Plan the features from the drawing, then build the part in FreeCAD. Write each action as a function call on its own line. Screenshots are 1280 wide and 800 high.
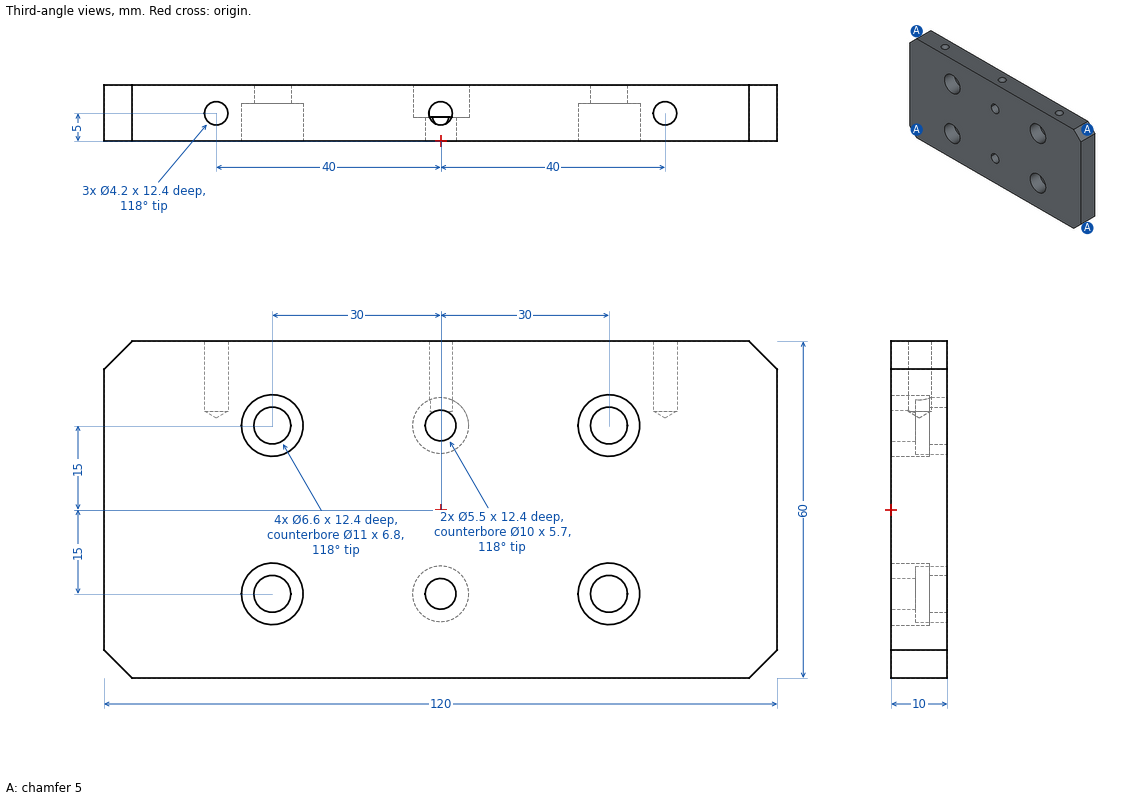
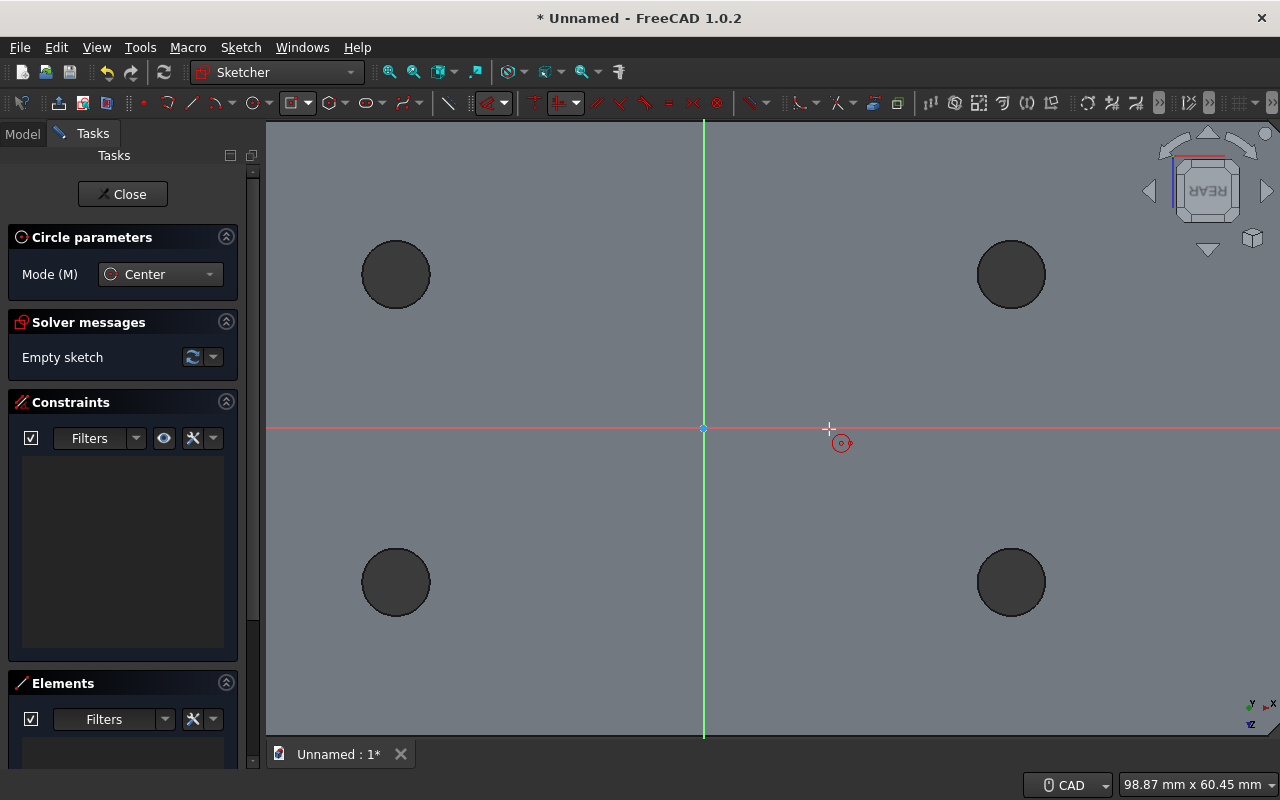
click(704, 582)
move(724, 562)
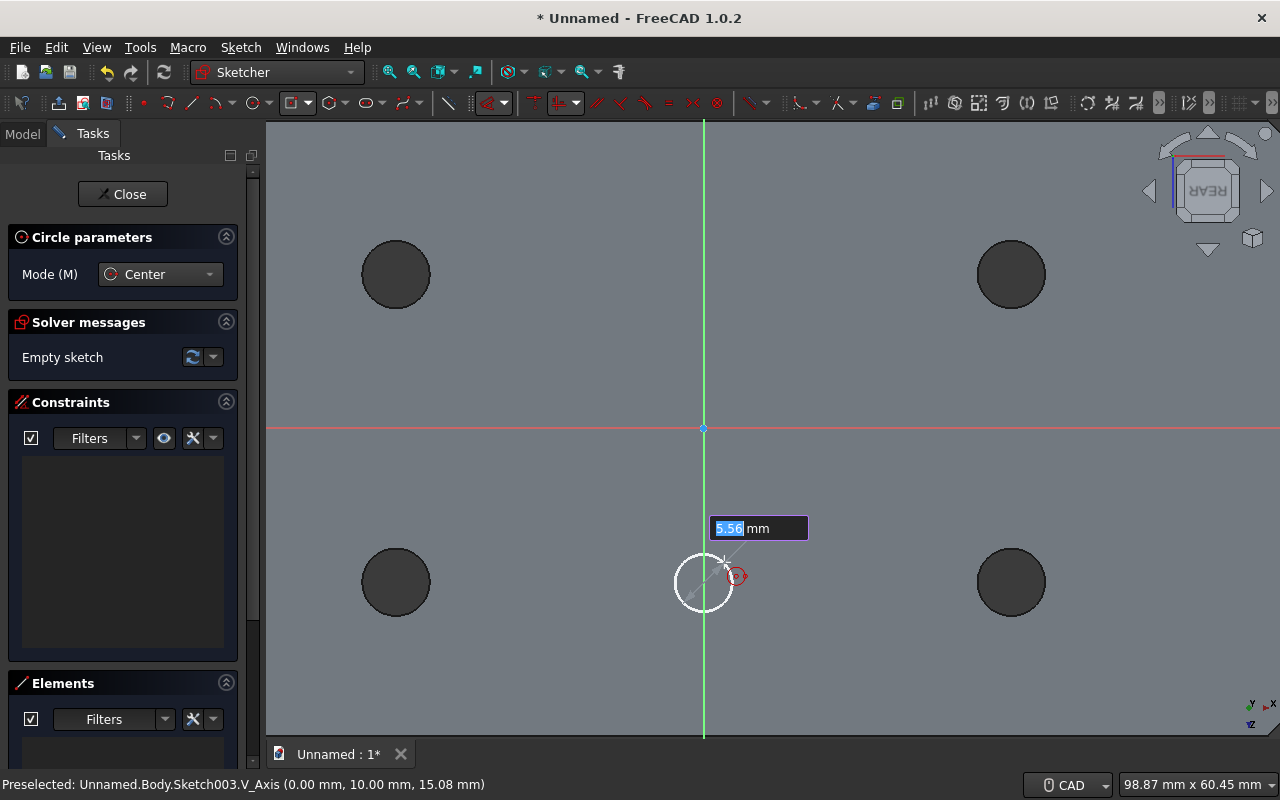
text(5.5)
key(Return)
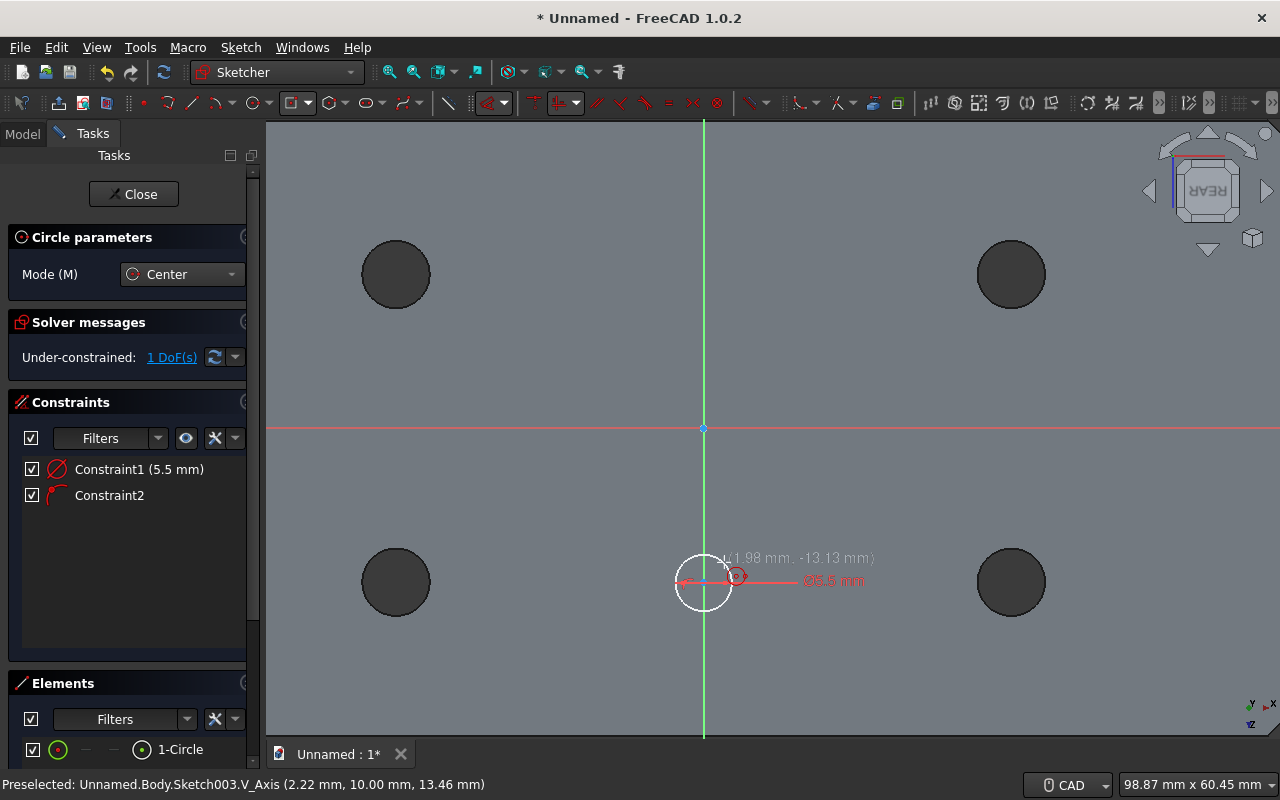
click(704, 275)
move(724, 255)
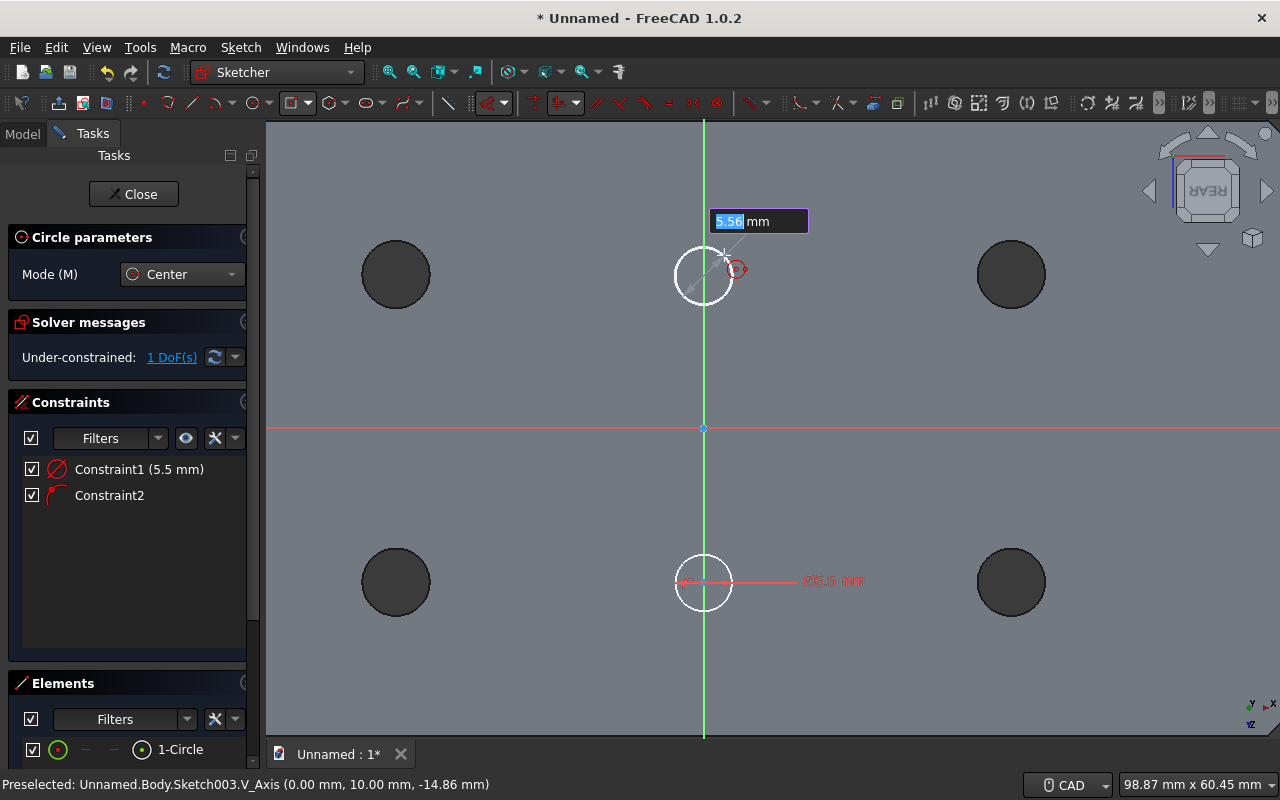
text(5.5)
key(Return)
key(Escape)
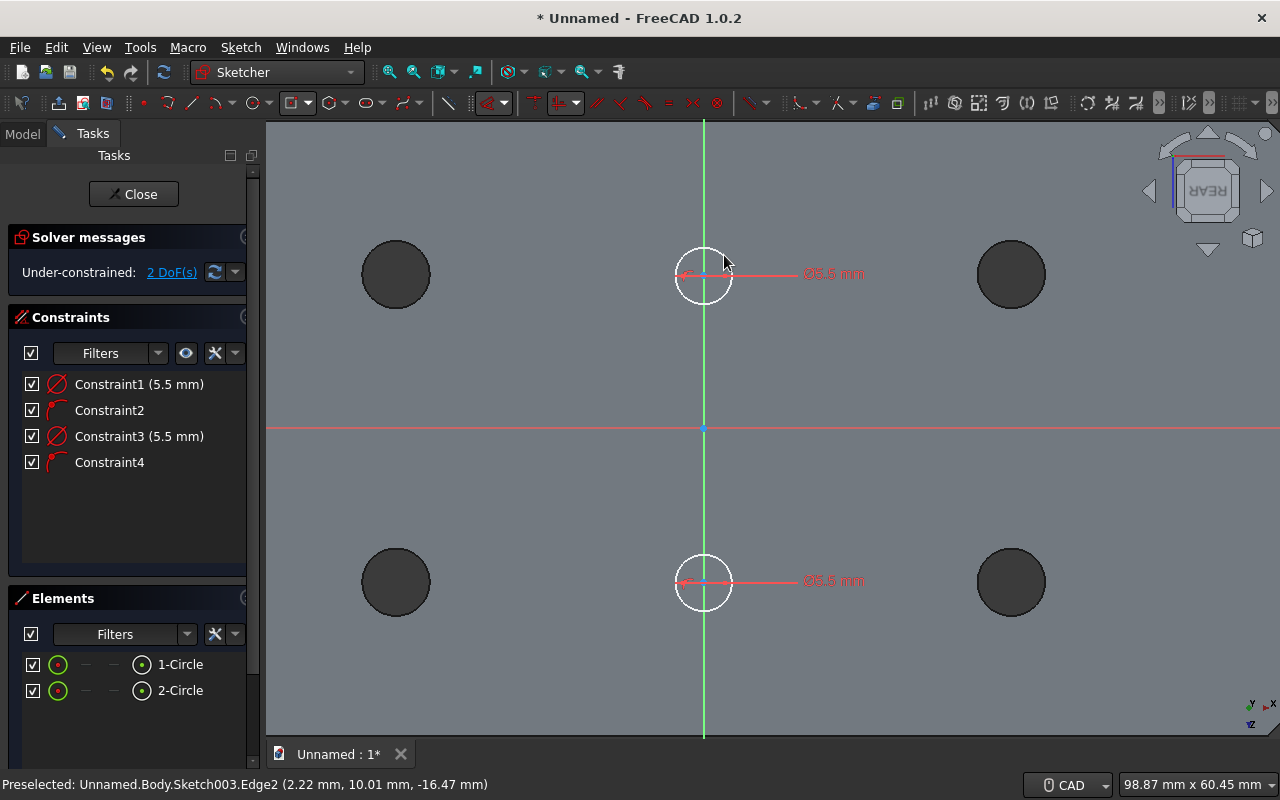
click(704, 583)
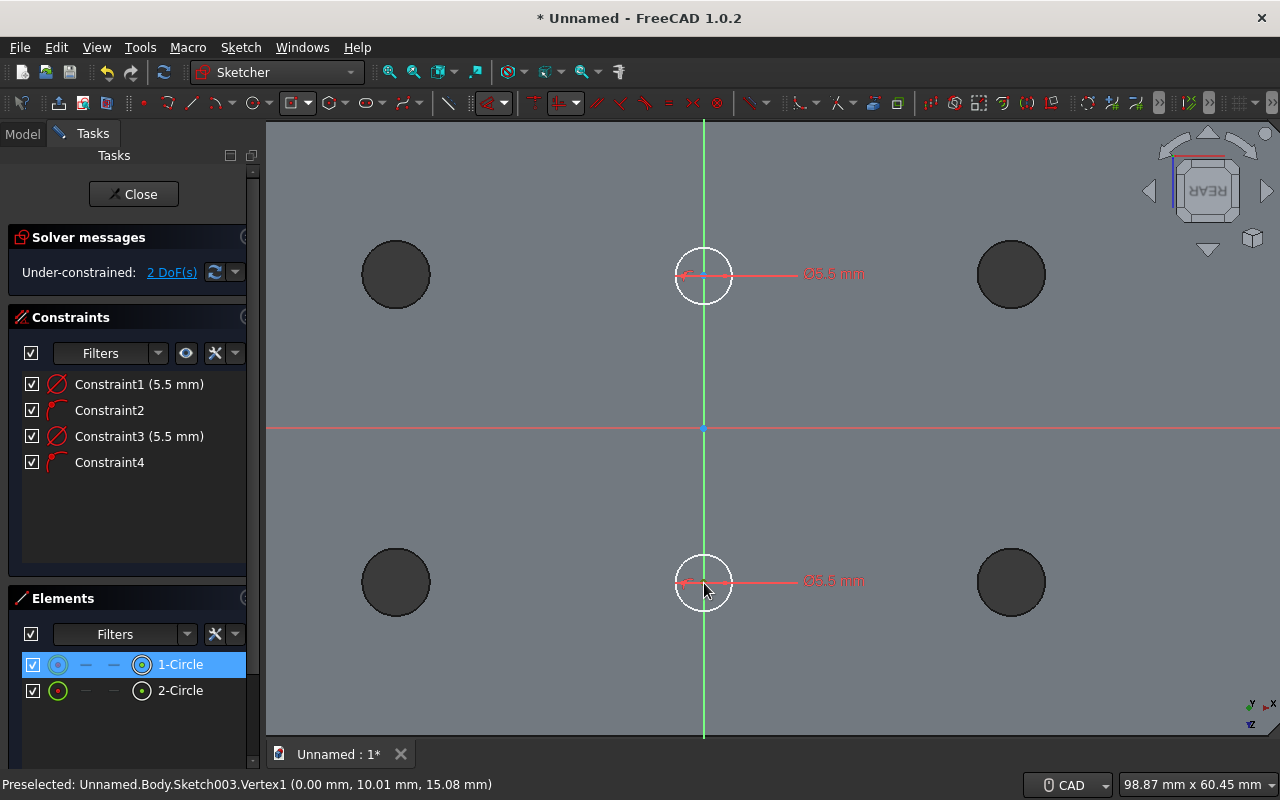
key(i)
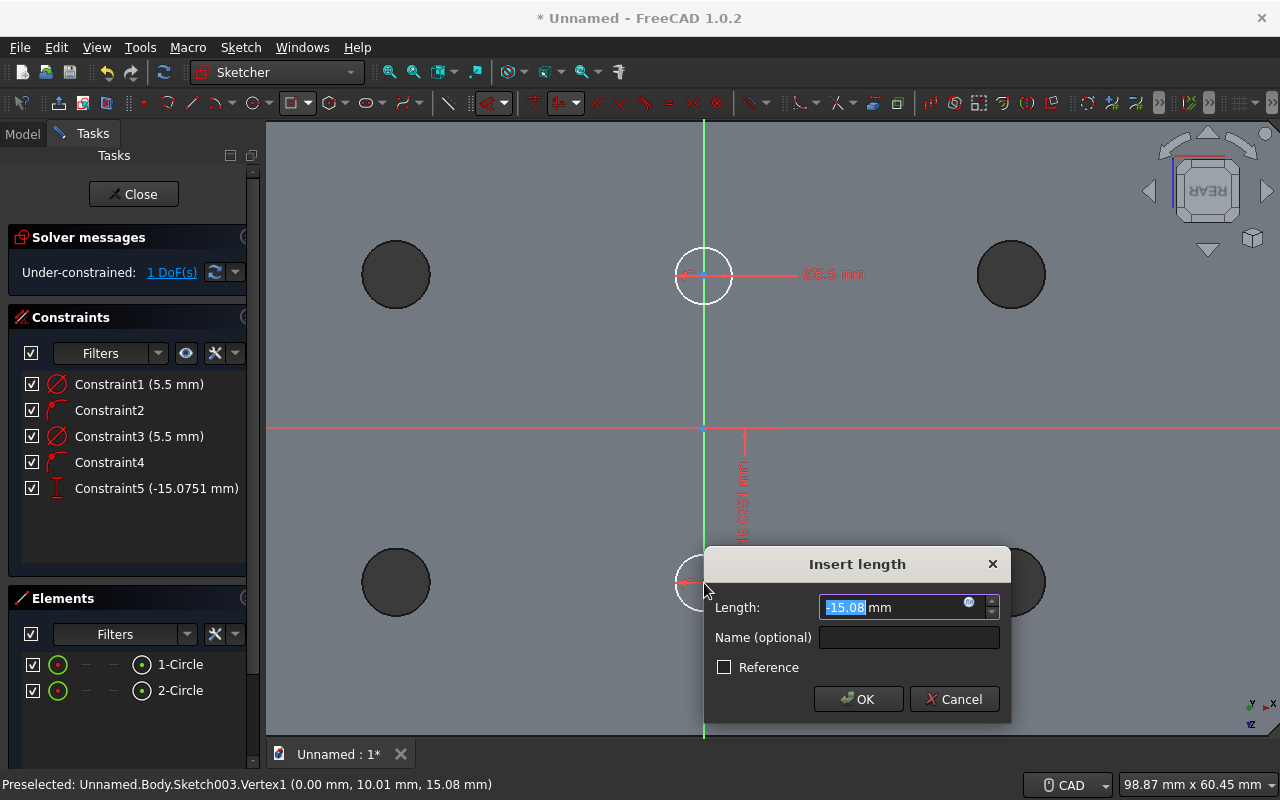
text(-15)
key(Return)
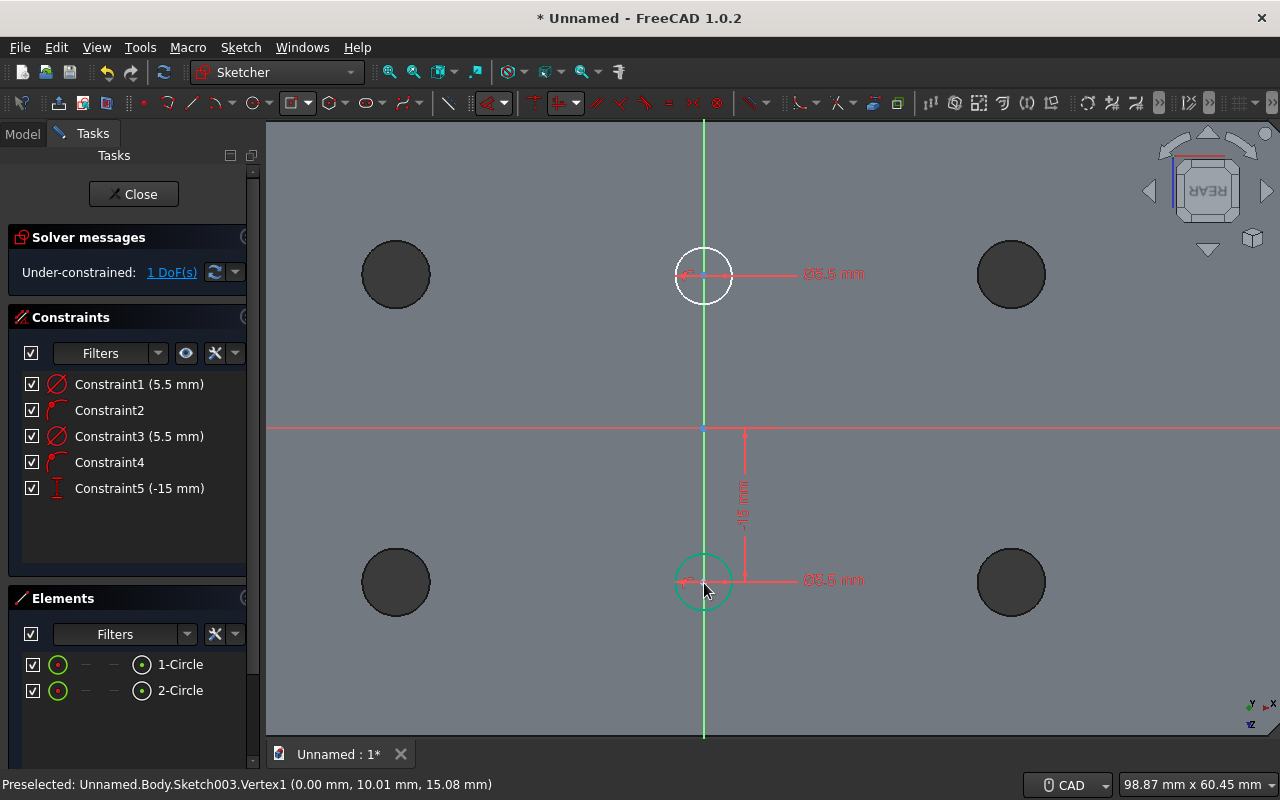
click(704, 276)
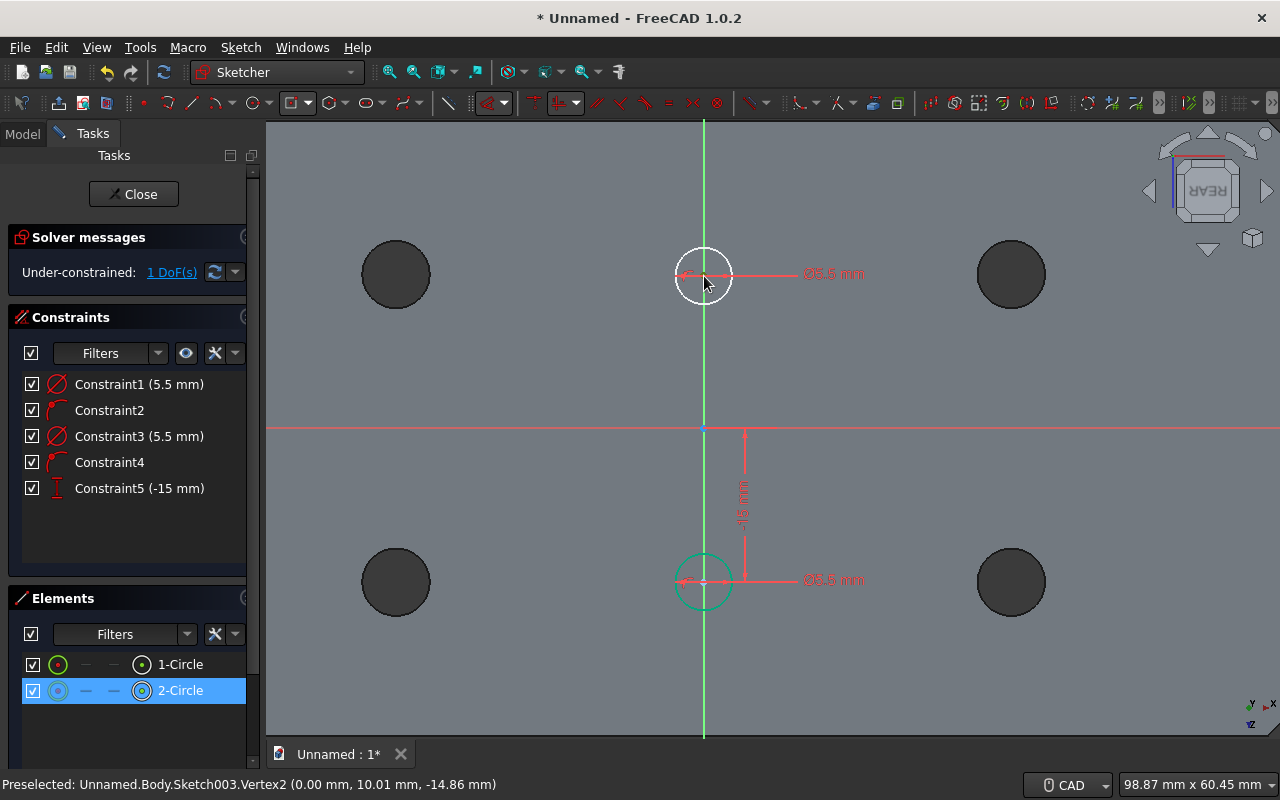
key(i)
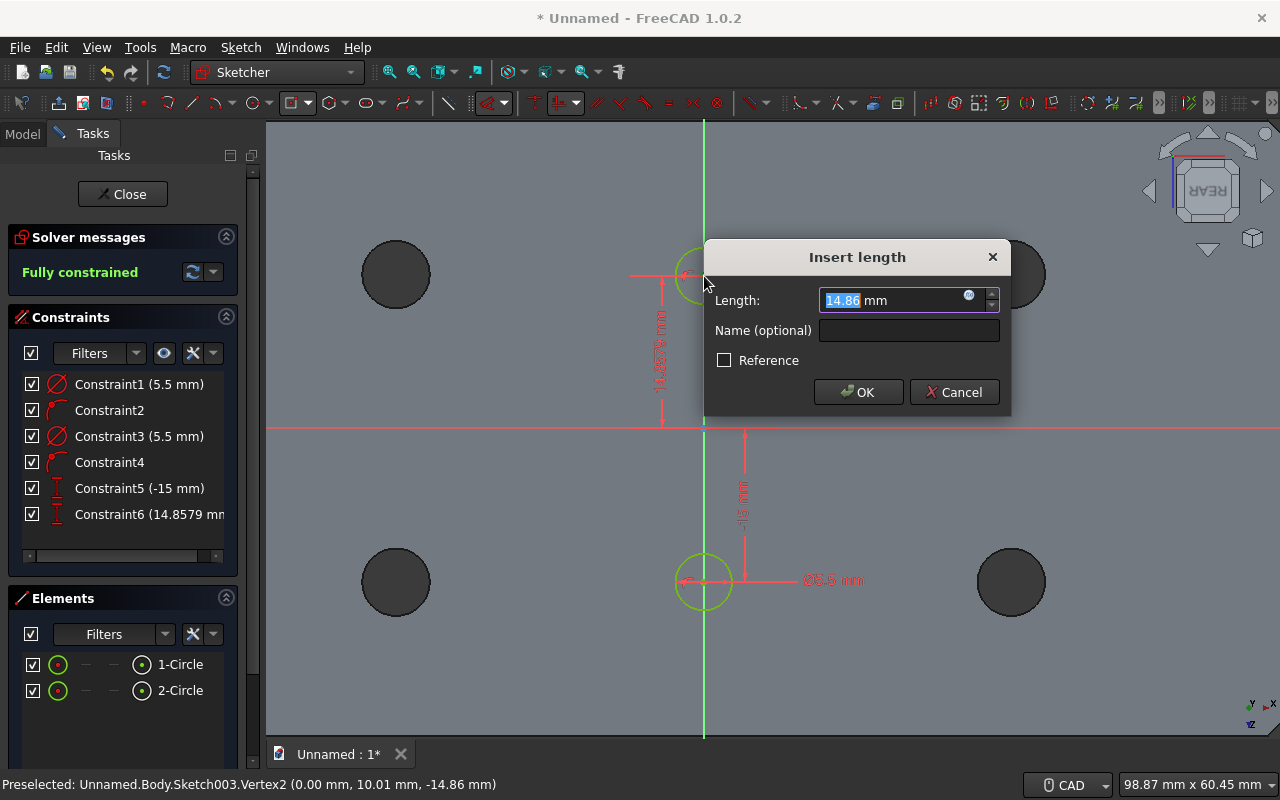
text(15)
key(Return)